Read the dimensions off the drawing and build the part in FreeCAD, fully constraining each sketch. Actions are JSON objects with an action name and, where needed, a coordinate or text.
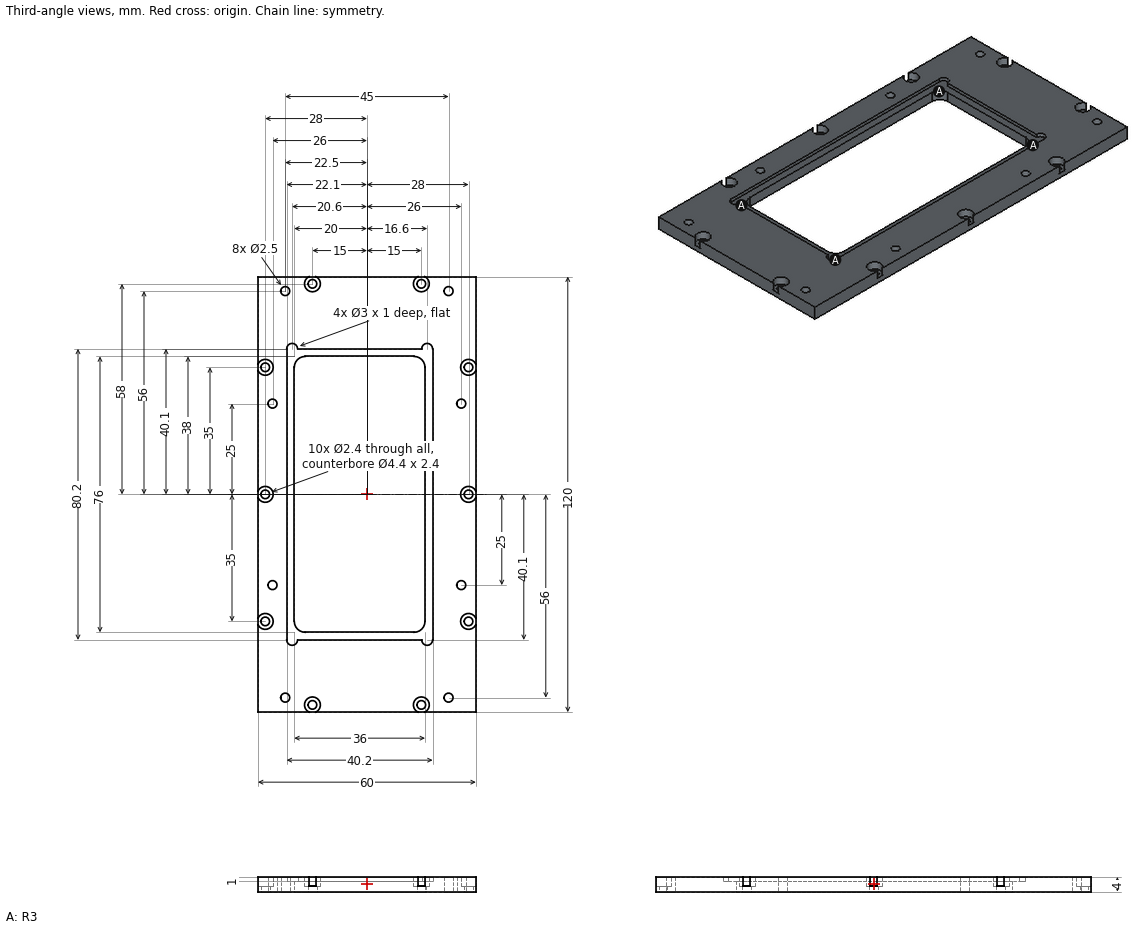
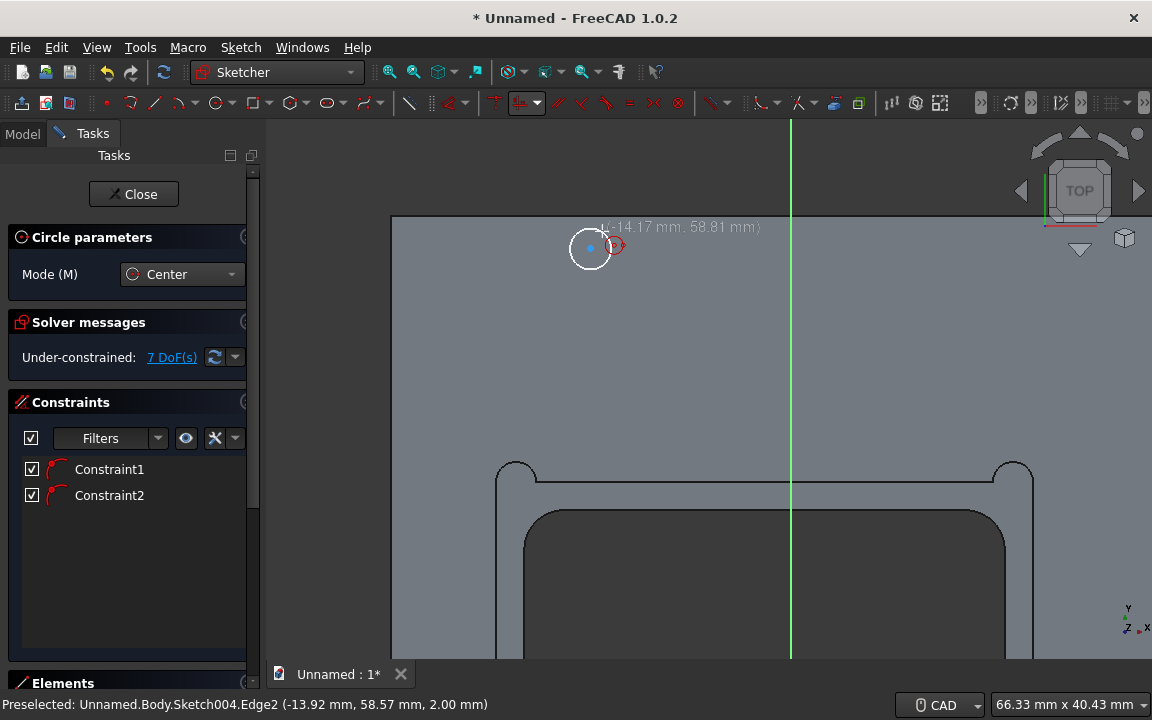
{"action": "scroll", "coordinate": [602, 230], "scroll_direction": "down", "scroll_amount": 8}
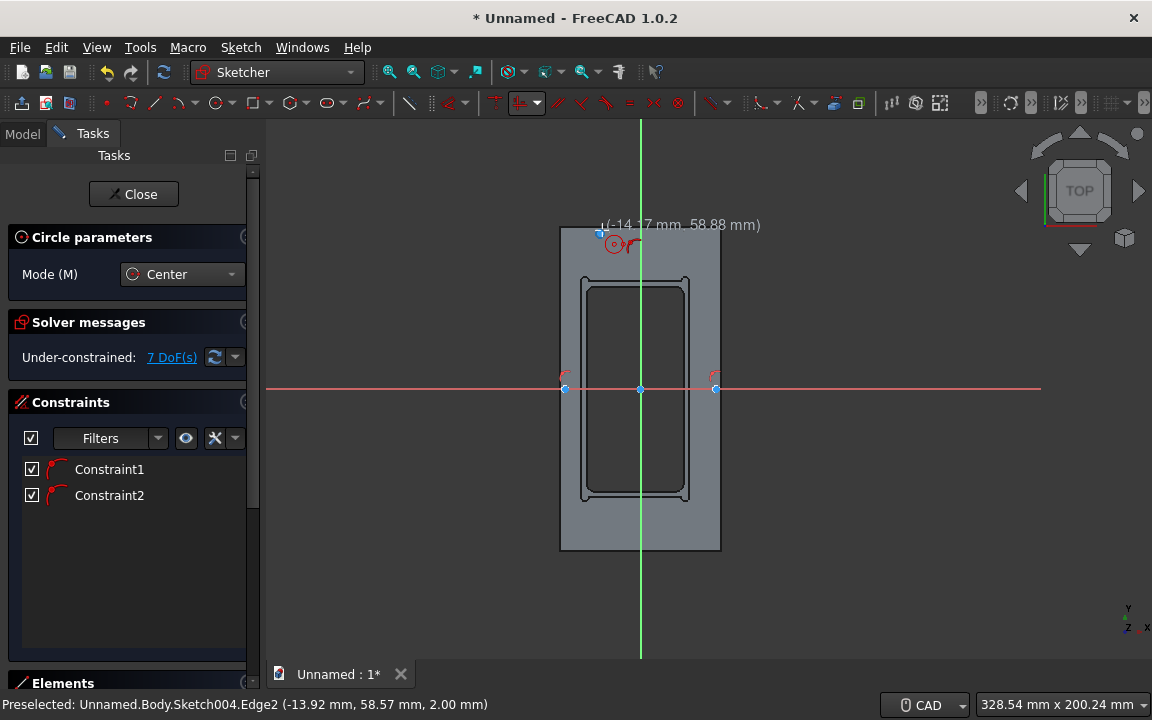
{"action": "scroll", "coordinate": [681, 233], "scroll_direction": "up", "scroll_amount": 10}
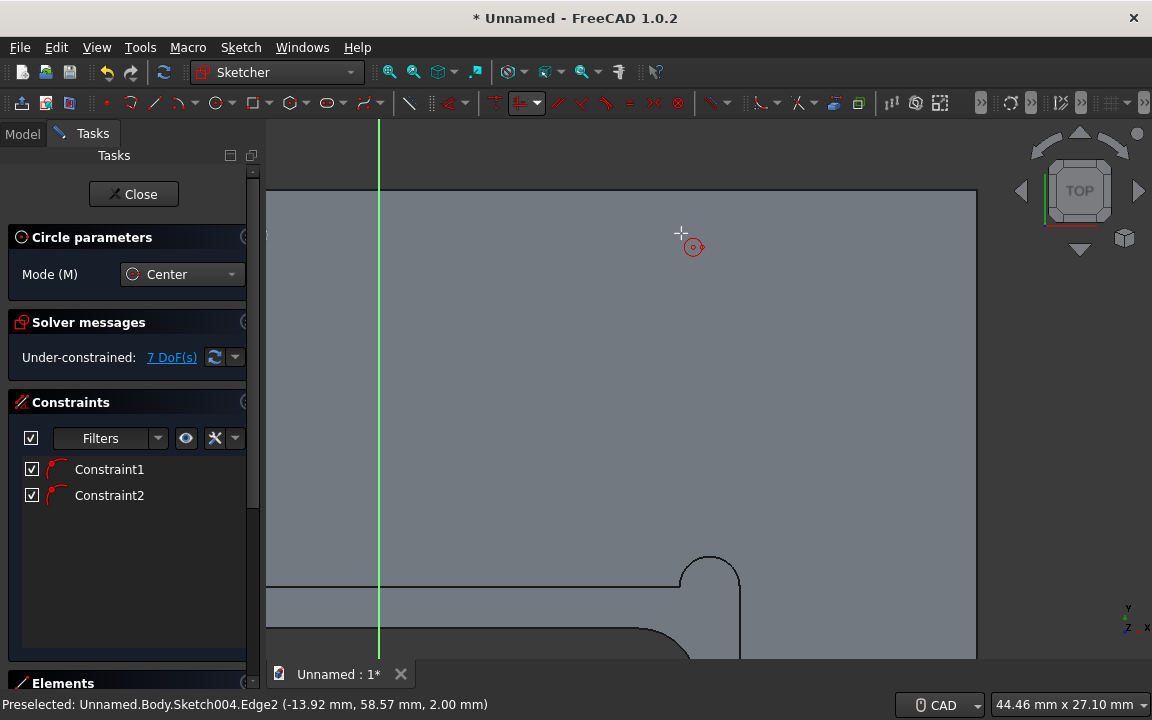
{"action": "scroll", "coordinate": [681, 233], "scroll_direction": "down", "scroll_amount": 10}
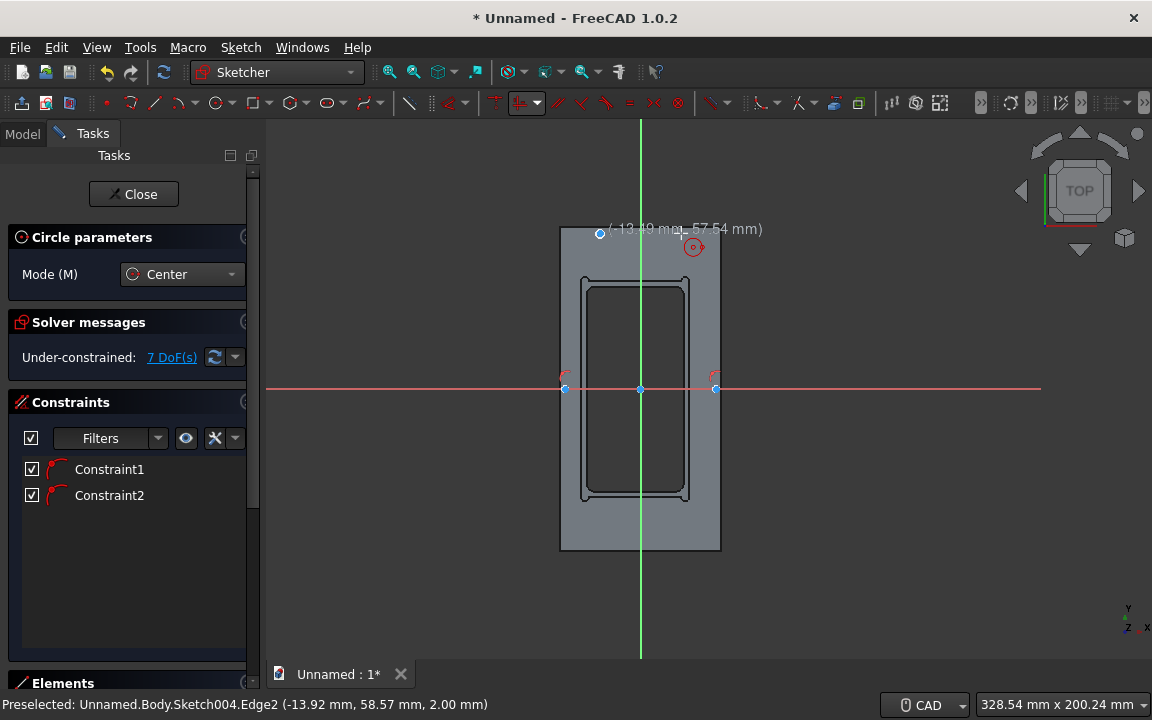
{"action": "left_click", "coordinate": [681, 233]}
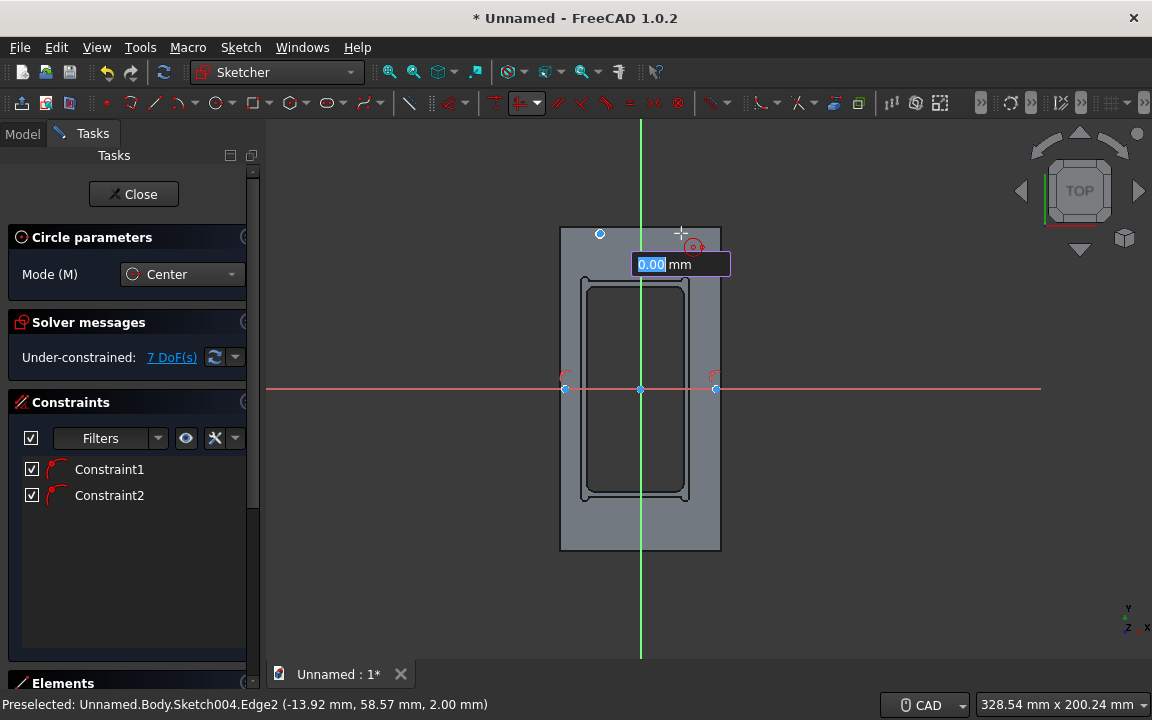
{"action": "scroll", "coordinate": [683, 230], "scroll_direction": "up", "scroll_amount": 8}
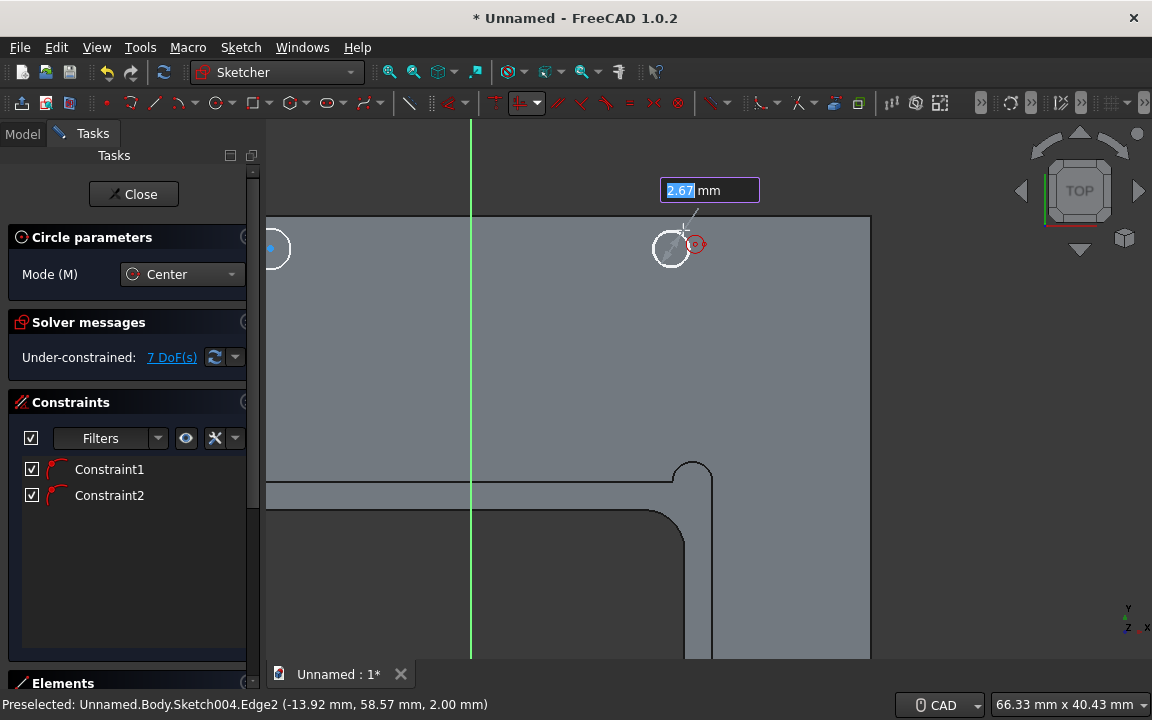
{"action": "left_click", "coordinate": [682, 231]}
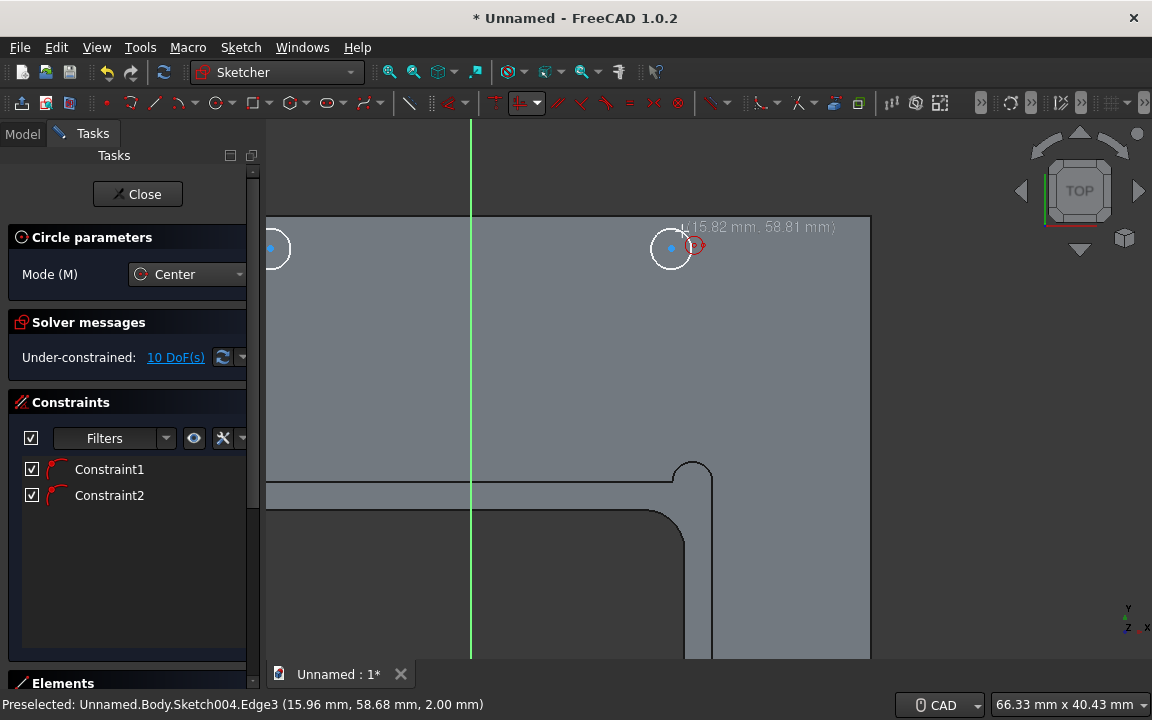
{"action": "scroll", "coordinate": [683, 230], "scroll_direction": "down", "scroll_amount": 8}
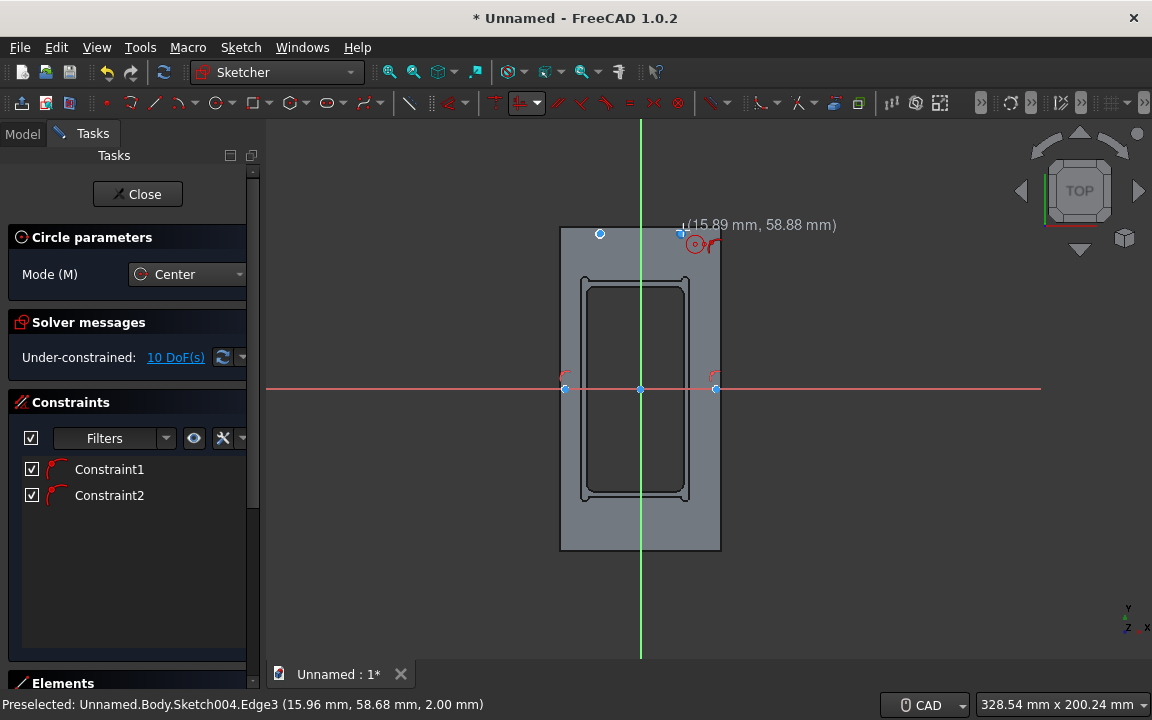
{"action": "scroll", "coordinate": [565, 295], "scroll_direction": "up", "scroll_amount": 10}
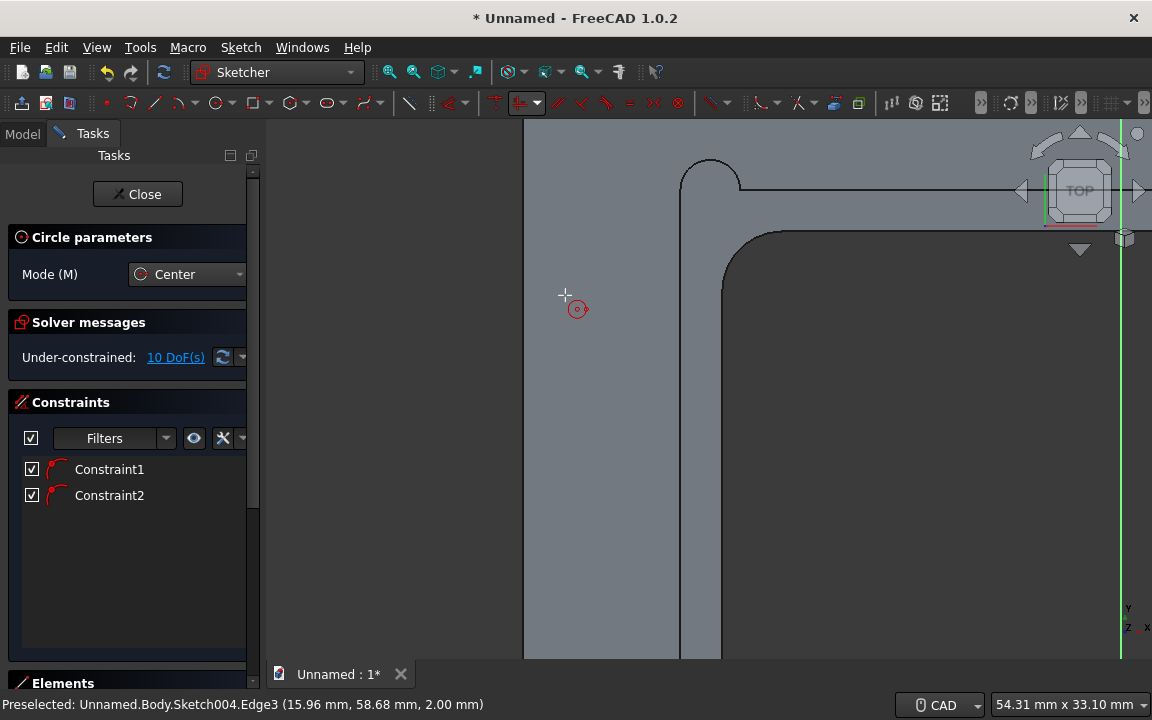
{"action": "scroll", "coordinate": [565, 295], "scroll_direction": "down", "scroll_amount": 10}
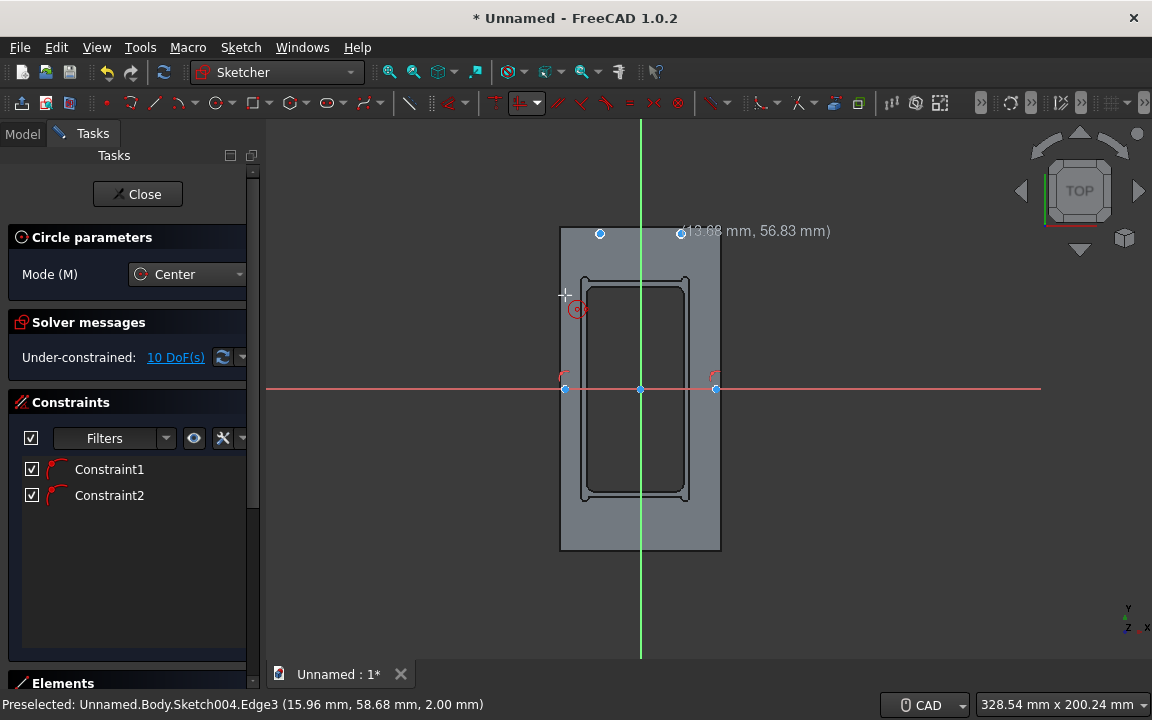
{"action": "left_click", "coordinate": [565, 295]}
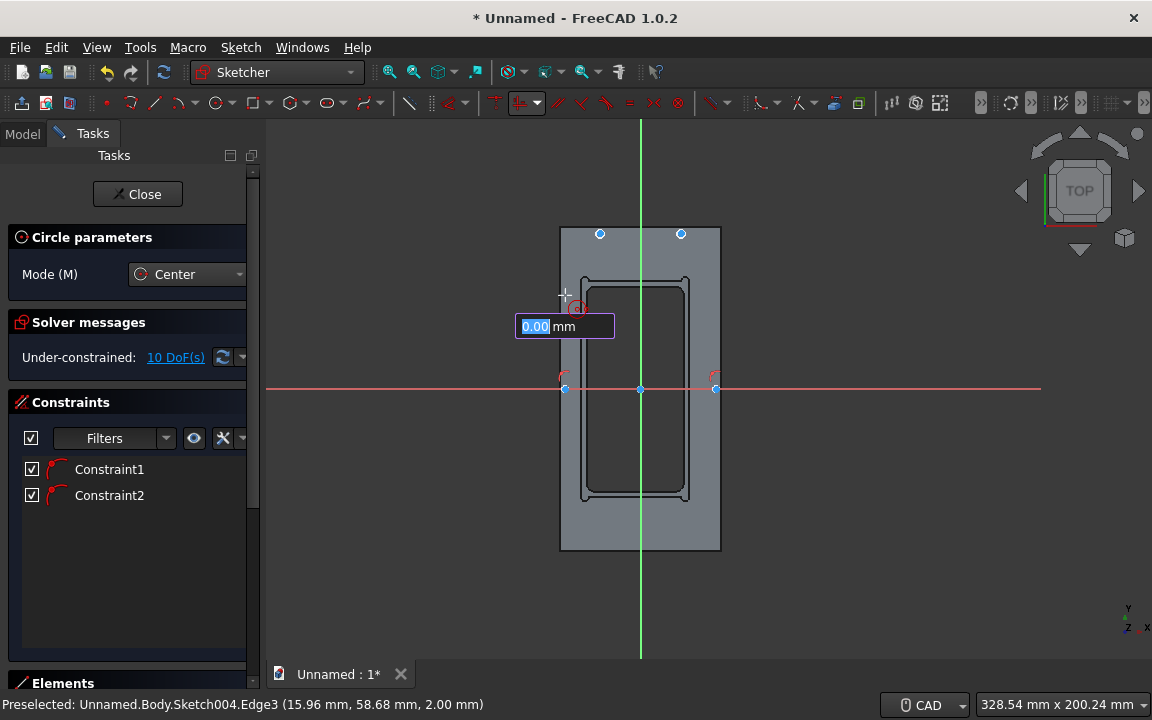
{"action": "scroll", "coordinate": [567, 292], "scroll_direction": "up", "scroll_amount": 8}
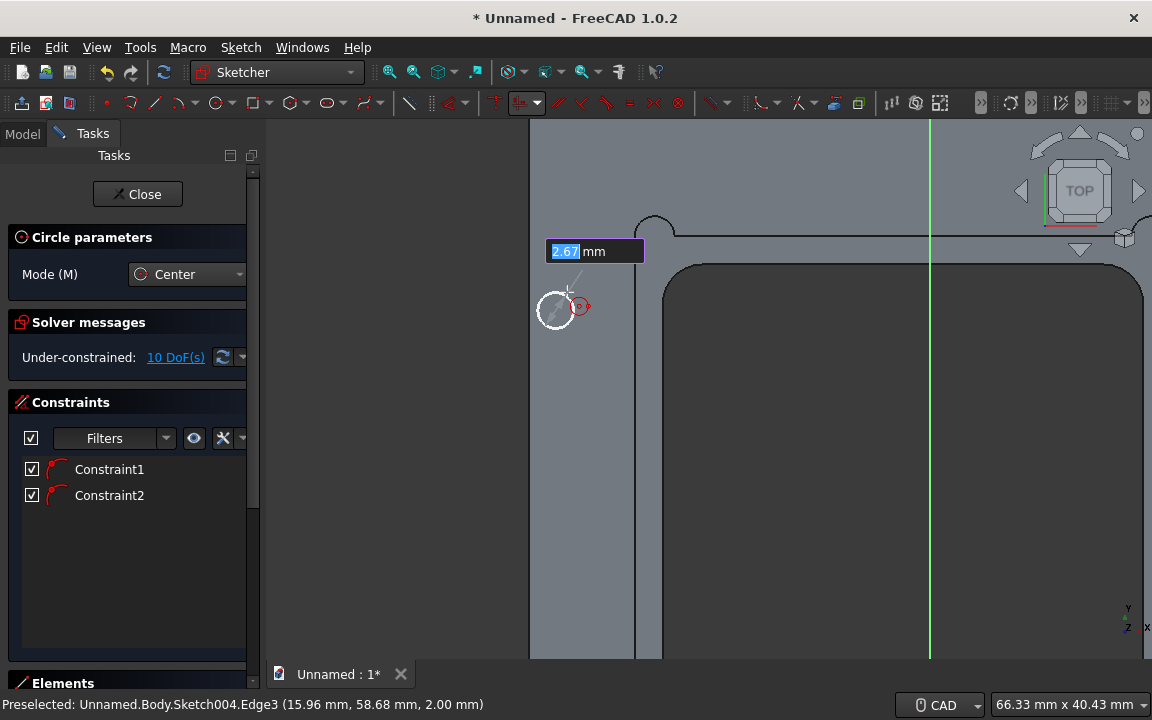
{"action": "left_click", "coordinate": [567, 293]}